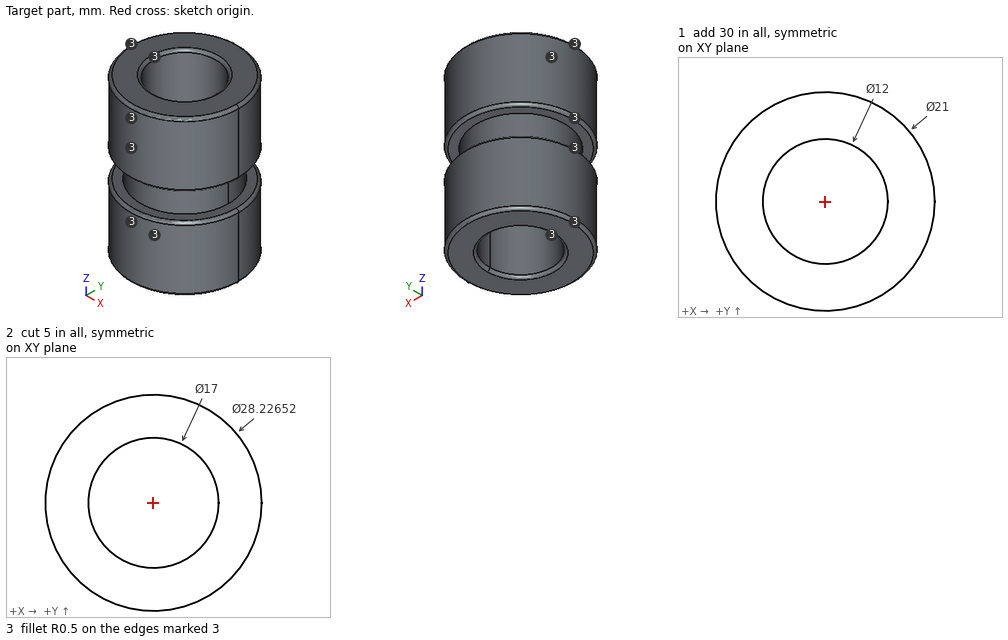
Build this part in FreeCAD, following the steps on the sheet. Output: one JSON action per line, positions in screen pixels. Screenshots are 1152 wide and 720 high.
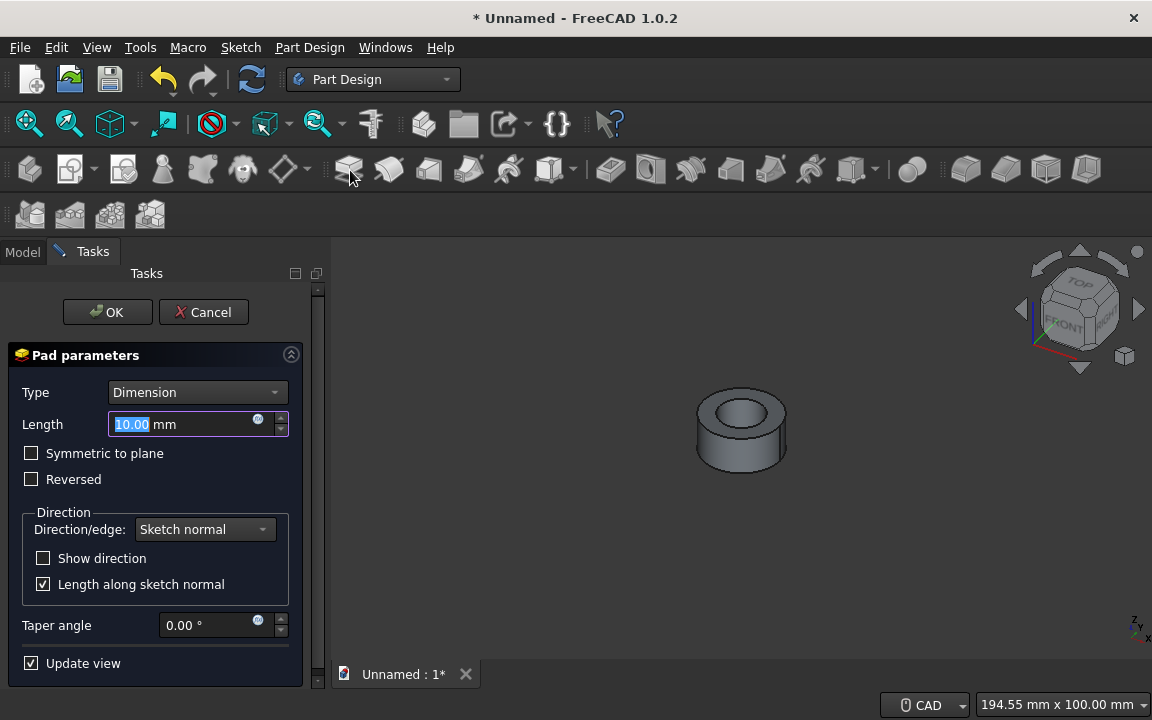
{"action": "type", "text": "30"}
{"action": "key", "text": "Tab"}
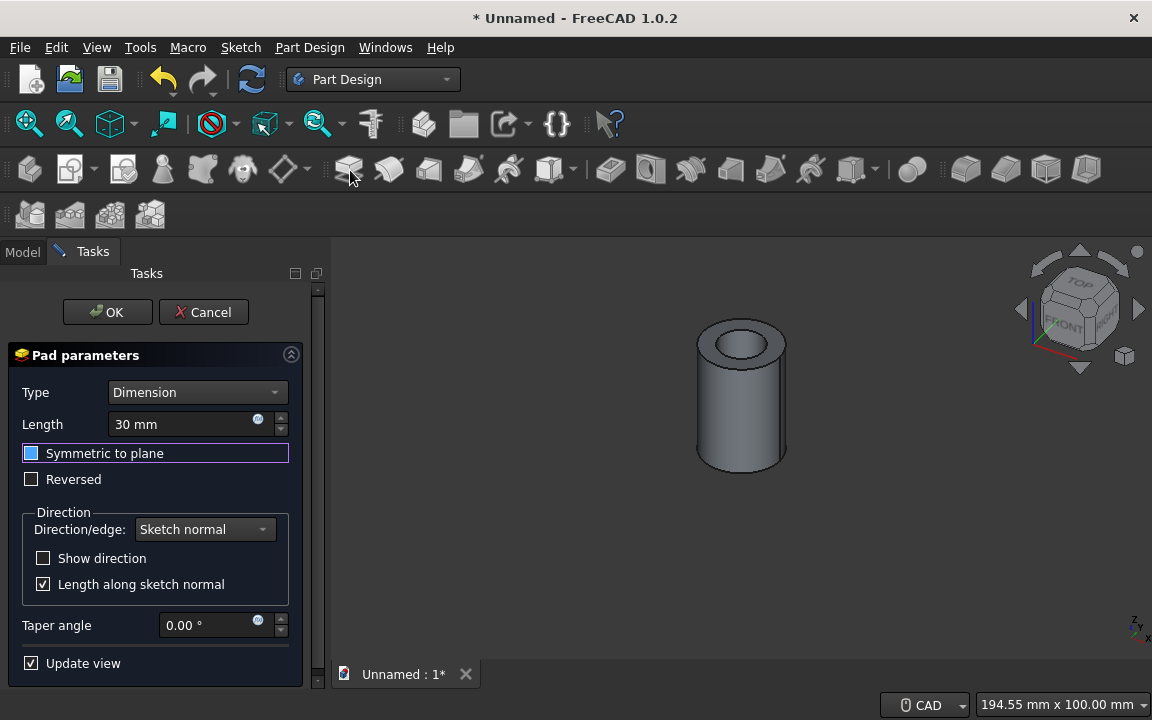
{"action": "left_click", "coordinate": [30, 453]}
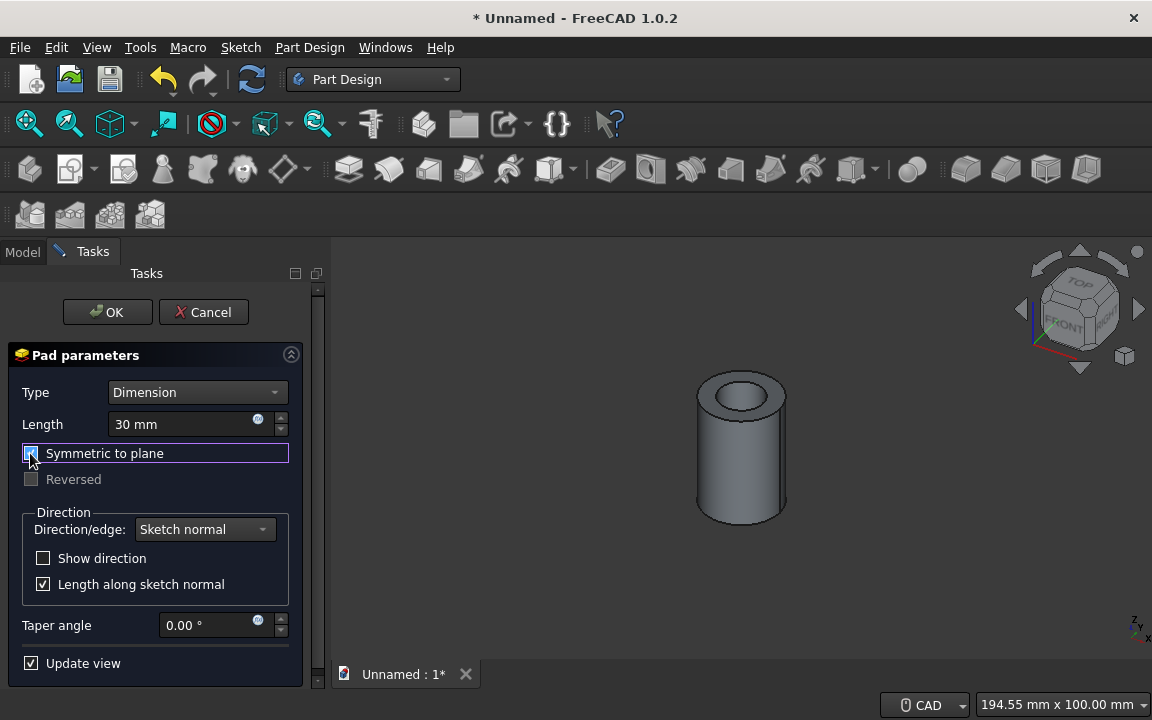
{"action": "left_click", "coordinate": [108, 312]}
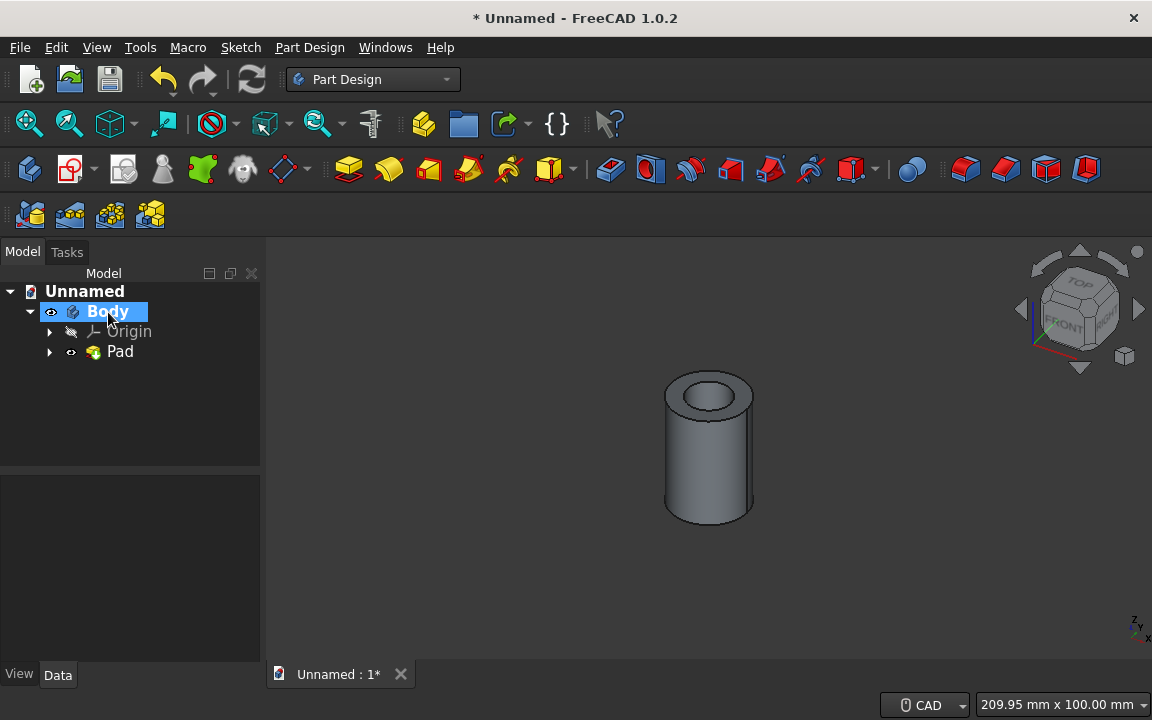
{"action": "key", "text": "v f"}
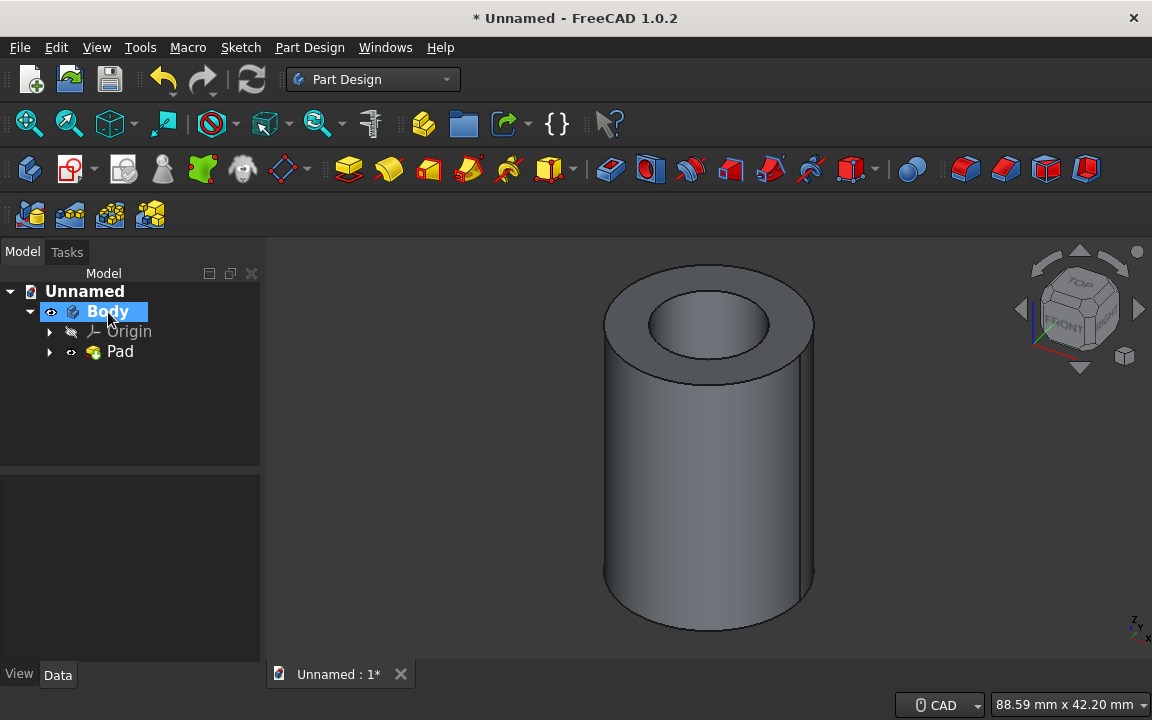
{"action": "left_click", "coordinate": [70, 170]}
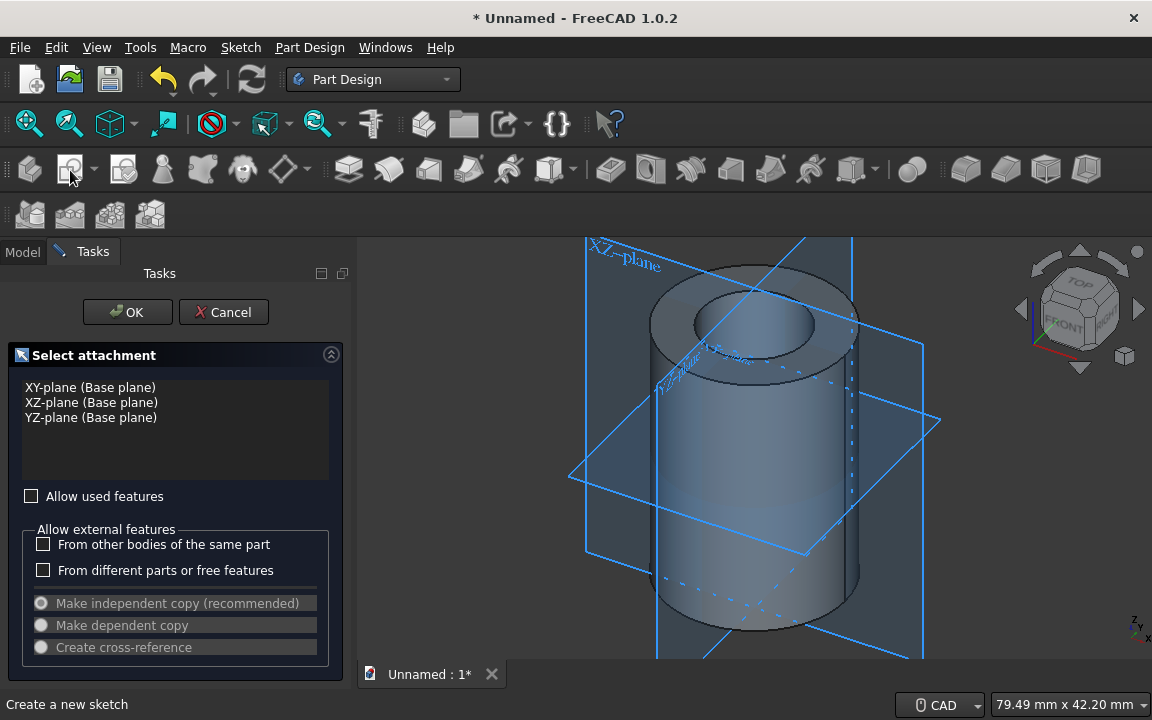
{"action": "left_click", "coordinate": [82, 388]}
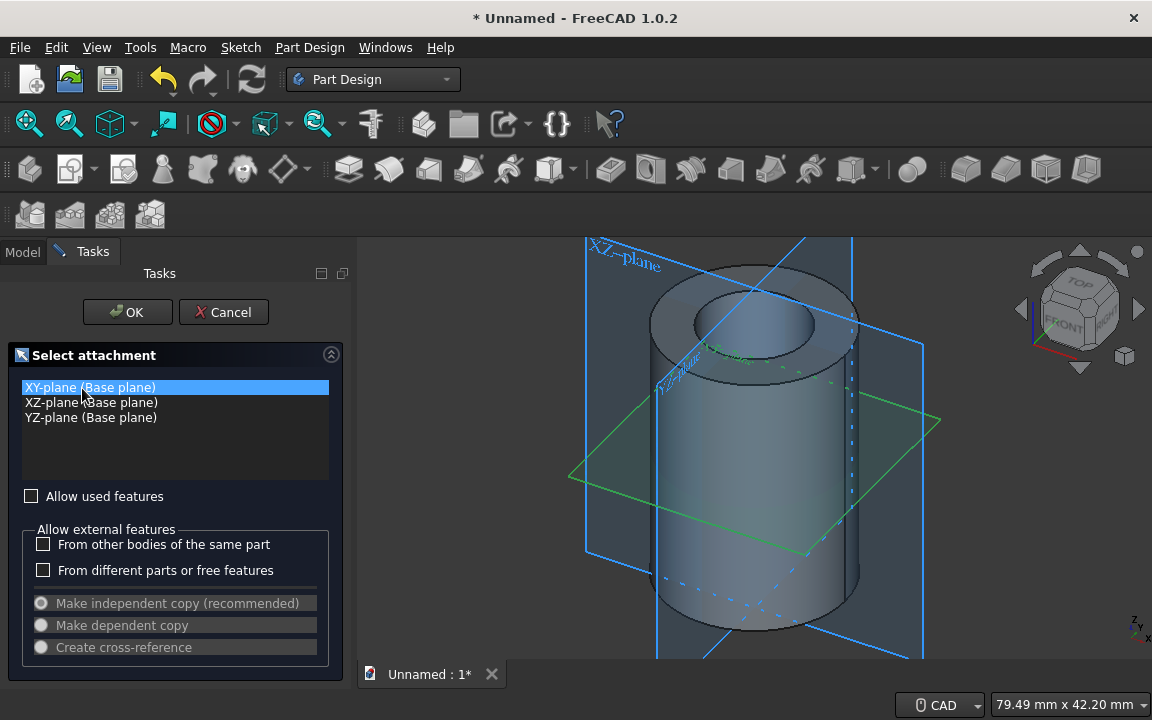
{"action": "left_click", "coordinate": [128, 312]}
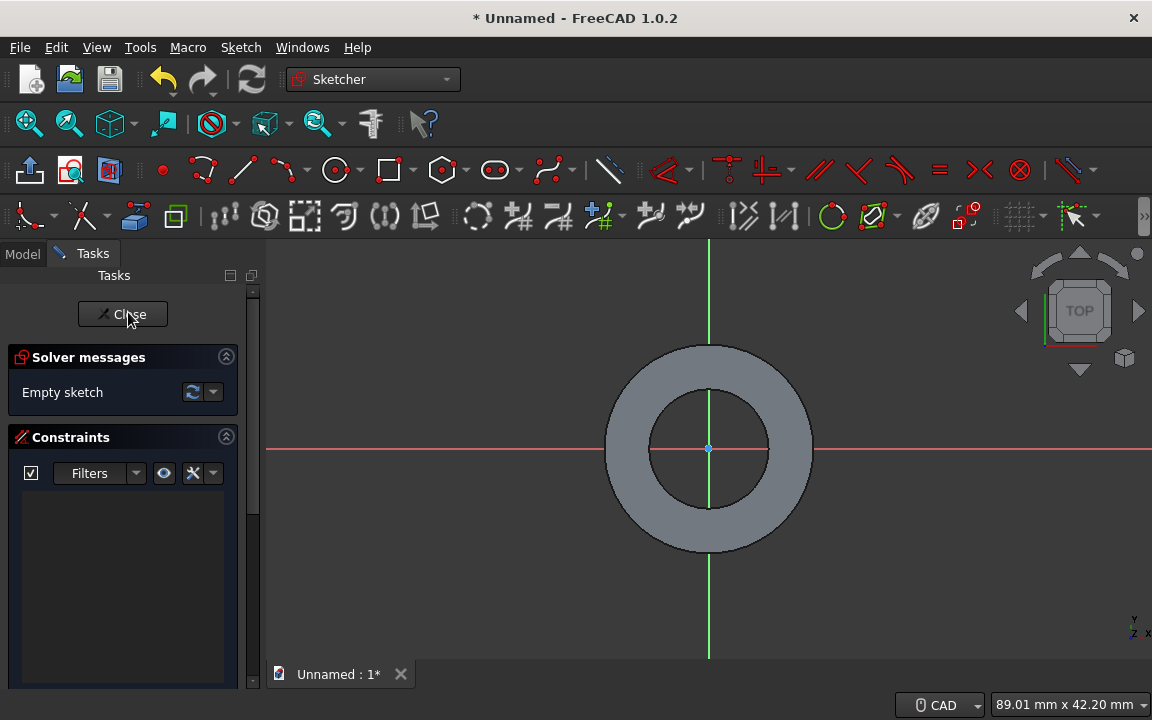
{"action": "key", "text": "q s"}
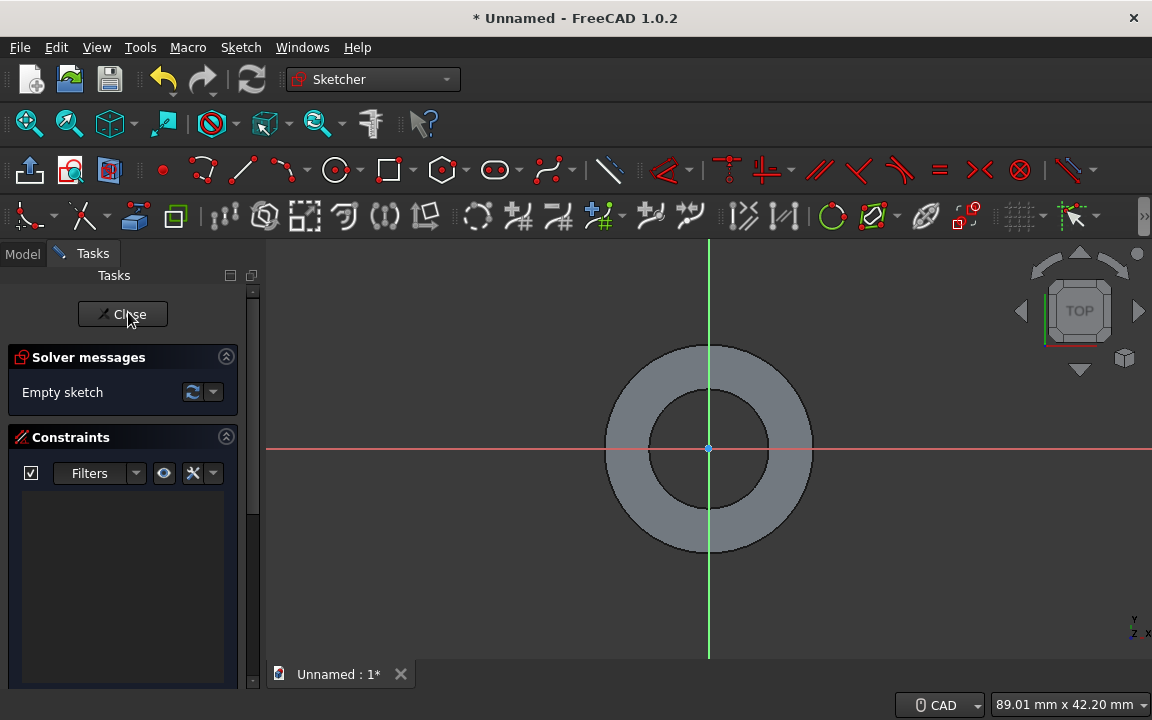
{"action": "left_click", "coordinate": [336, 170]}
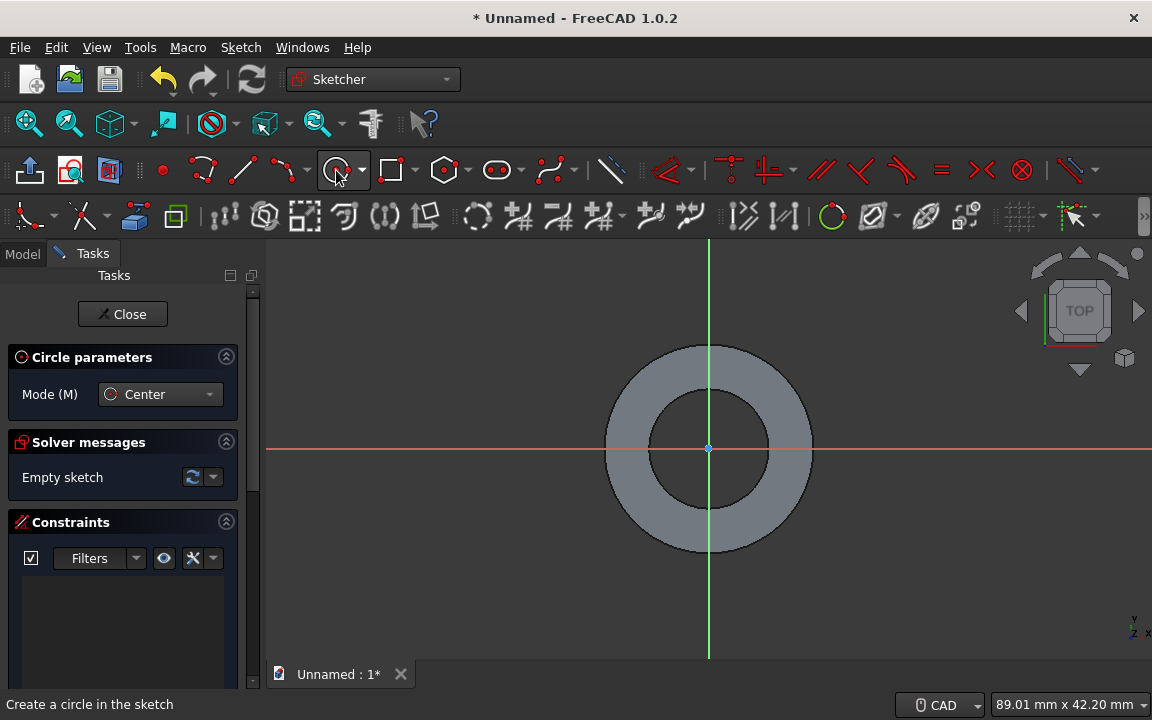
{"action": "left_click", "coordinate": [709, 449]}
{"action": "mouse_move", "coordinate": [808, 350]}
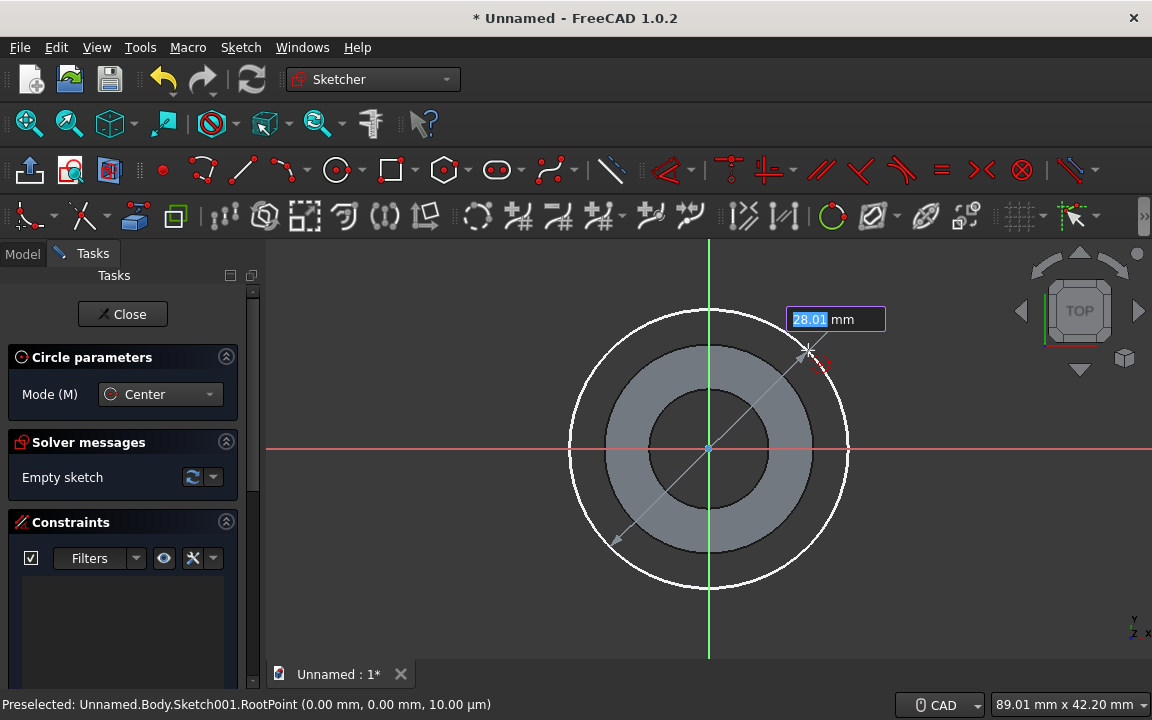
{"action": "type", "text": "28.22652"}
{"action": "key", "text": "Return"}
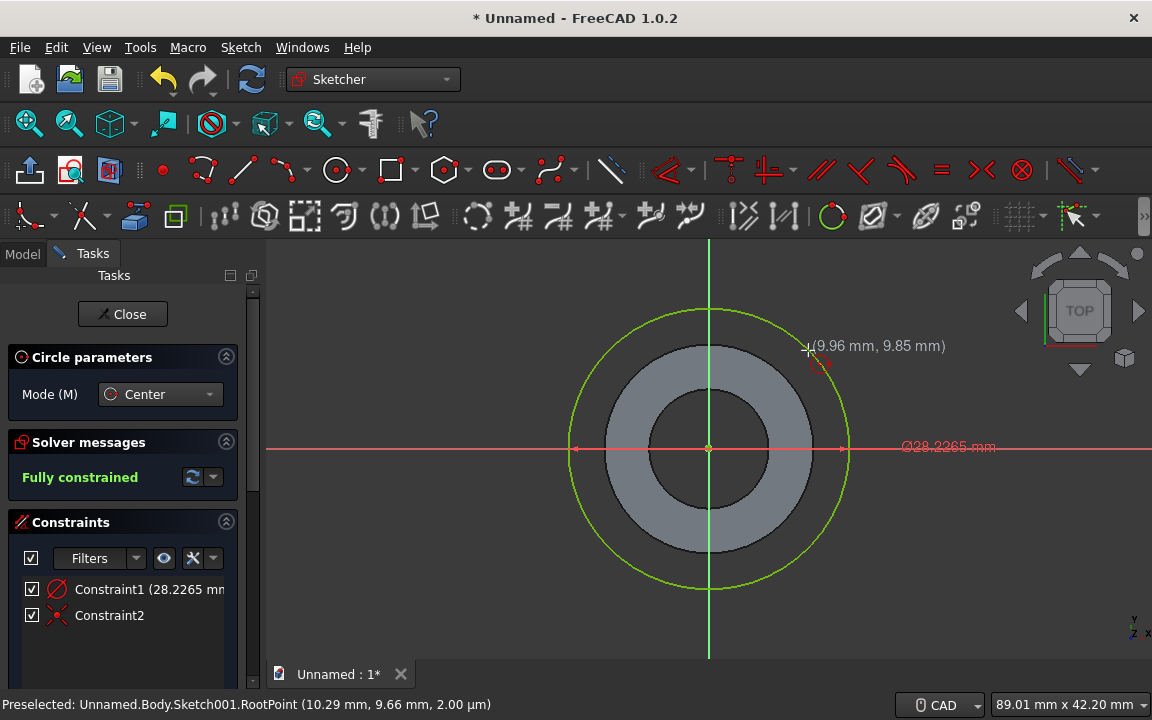
{"action": "left_click", "coordinate": [709, 449]}
{"action": "mouse_move", "coordinate": [769, 389]}